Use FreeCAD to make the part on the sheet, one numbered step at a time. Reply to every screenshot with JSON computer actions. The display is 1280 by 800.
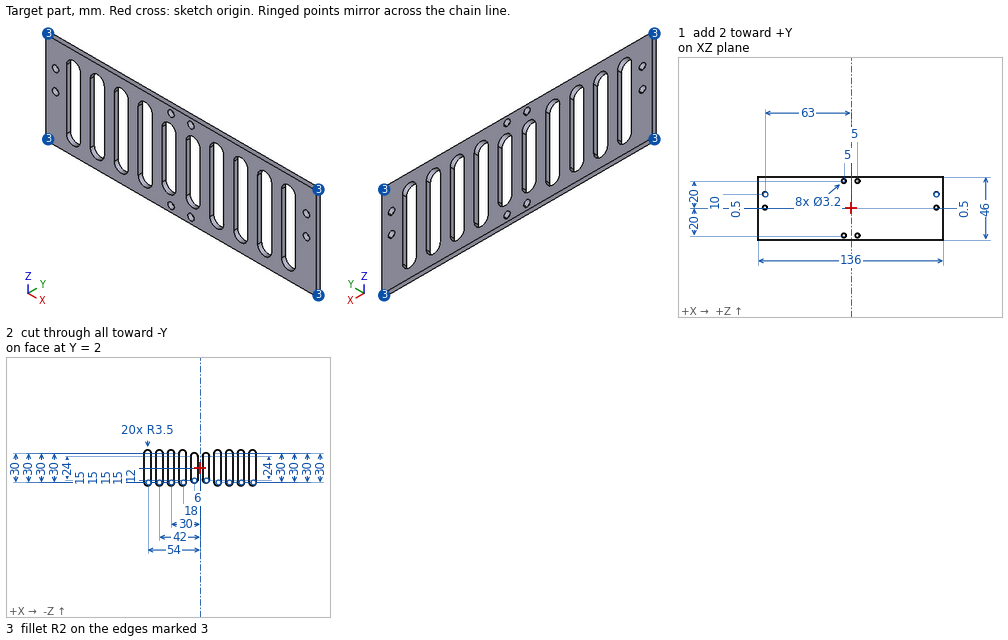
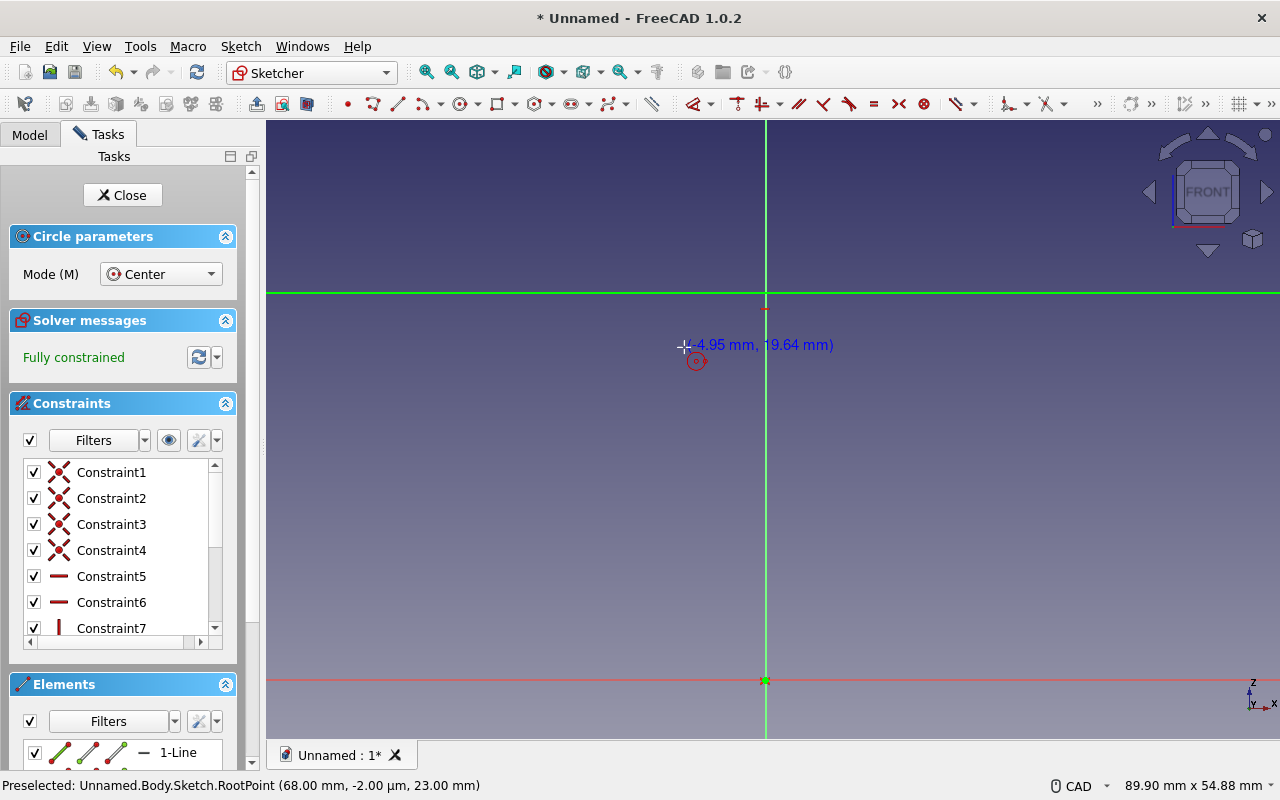
{"action": "scroll", "coordinate": [684, 347], "scroll_direction": "down", "scroll_amount": 7}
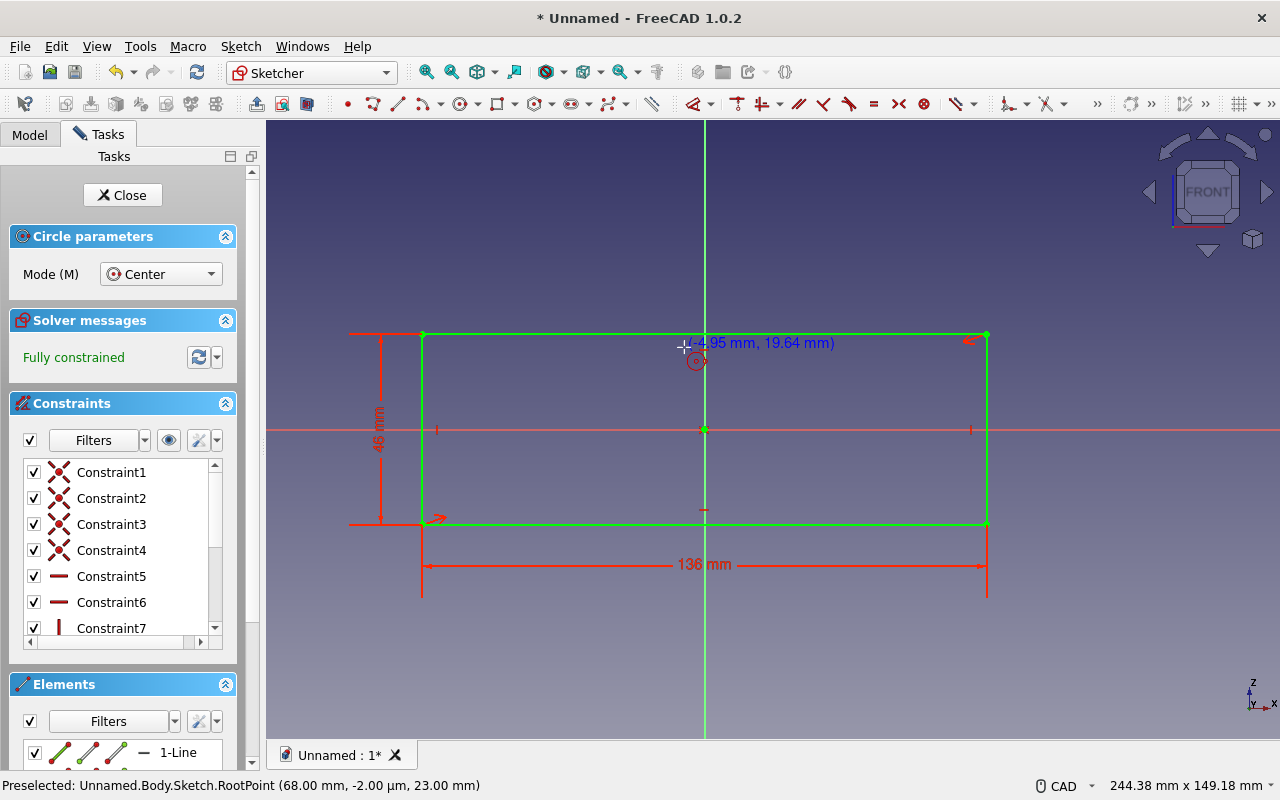
{"action": "scroll", "coordinate": [684, 347], "scroll_direction": "up", "scroll_amount": 2}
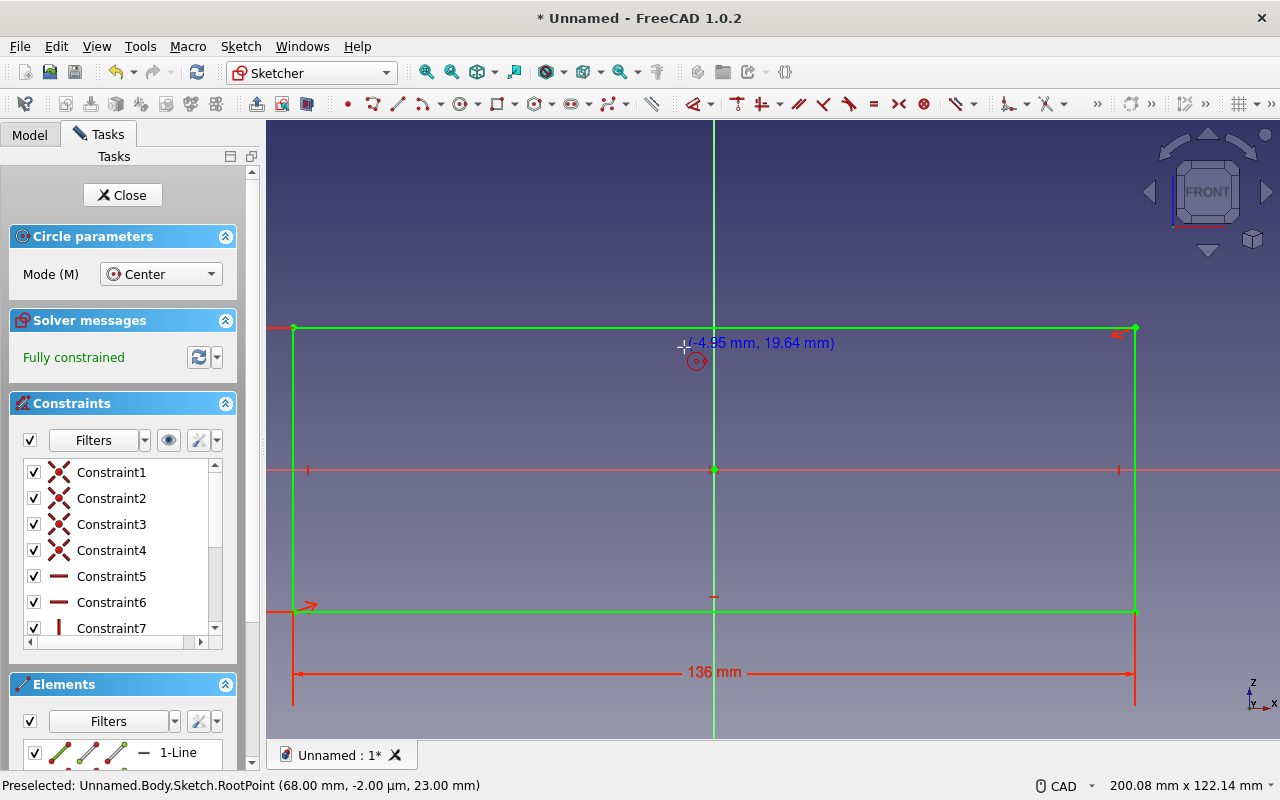
{"action": "left_click", "coordinate": [683, 346]}
{"action": "mouse_move", "coordinate": [690, 353]}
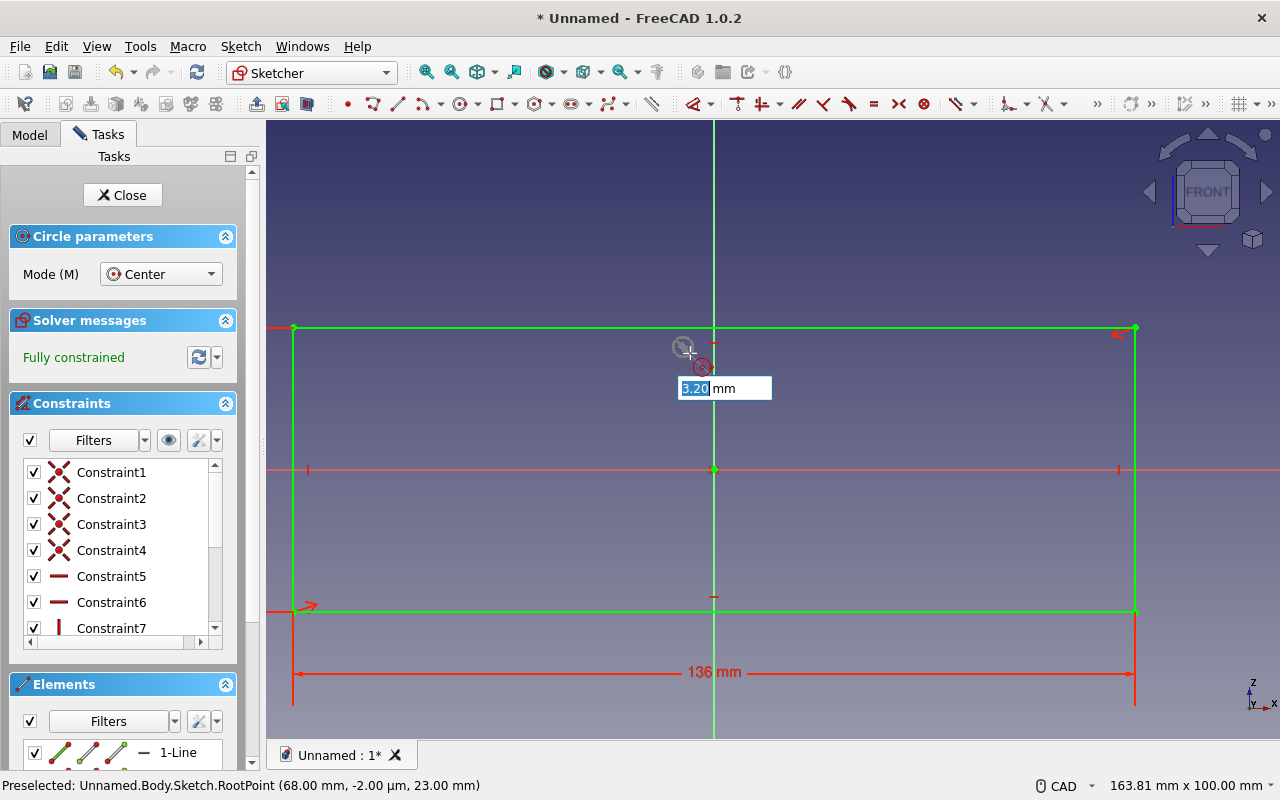
{"action": "type", "text": "3.2"}
{"action": "key", "text": "Return"}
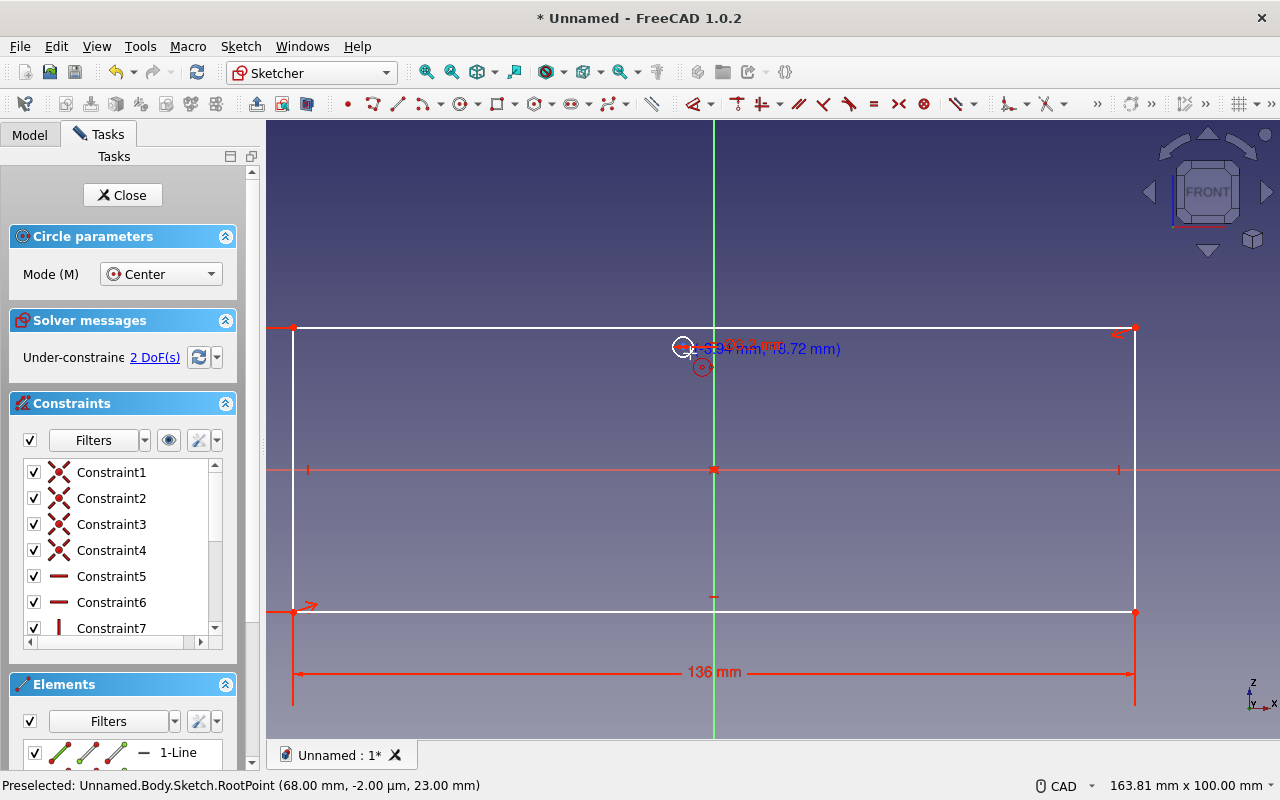
{"action": "scroll", "coordinate": [324, 405], "scroll_direction": "up", "scroll_amount": 5}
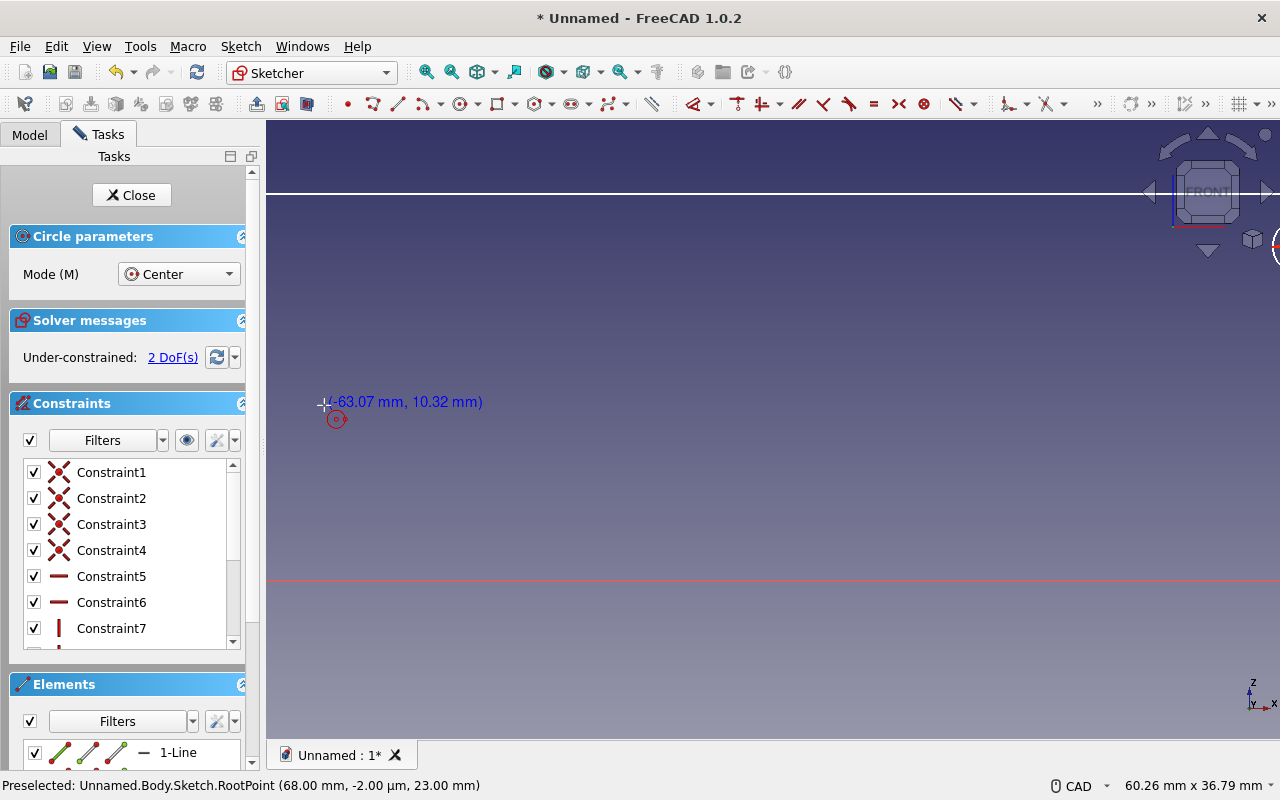
{"action": "scroll", "coordinate": [482, 380], "scroll_direction": "down", "scroll_amount": 7}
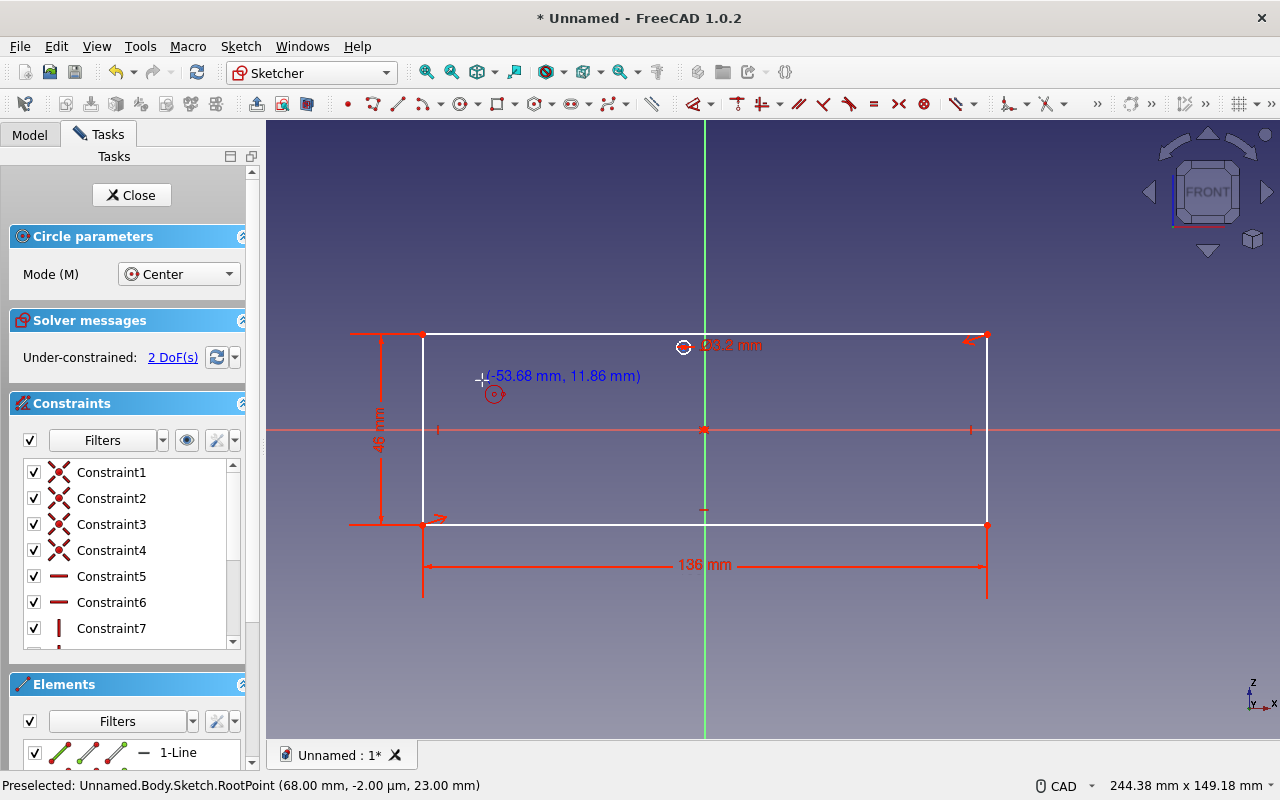
{"action": "left_click", "coordinate": [443, 386]}
{"action": "mouse_move", "coordinate": [448, 382]}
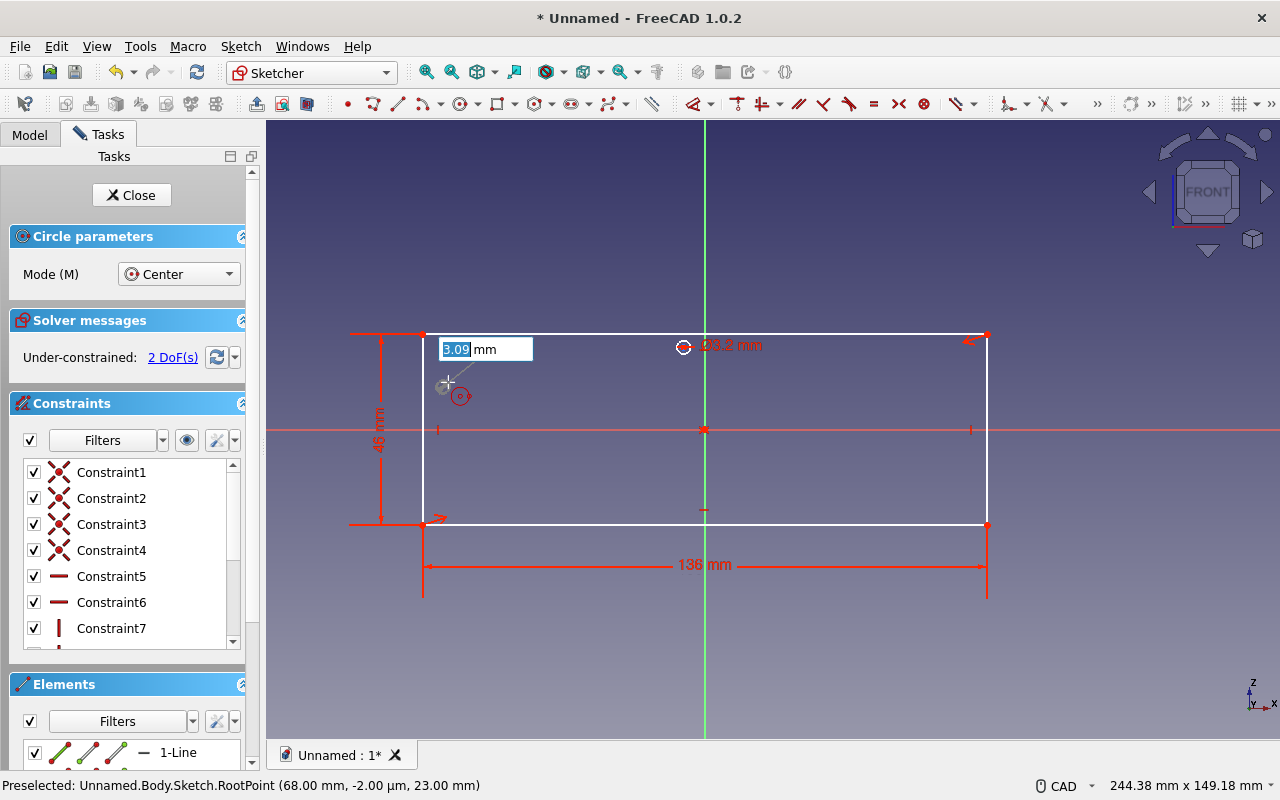
{"action": "type", "text": "3.2"}
{"action": "key", "text": "Return"}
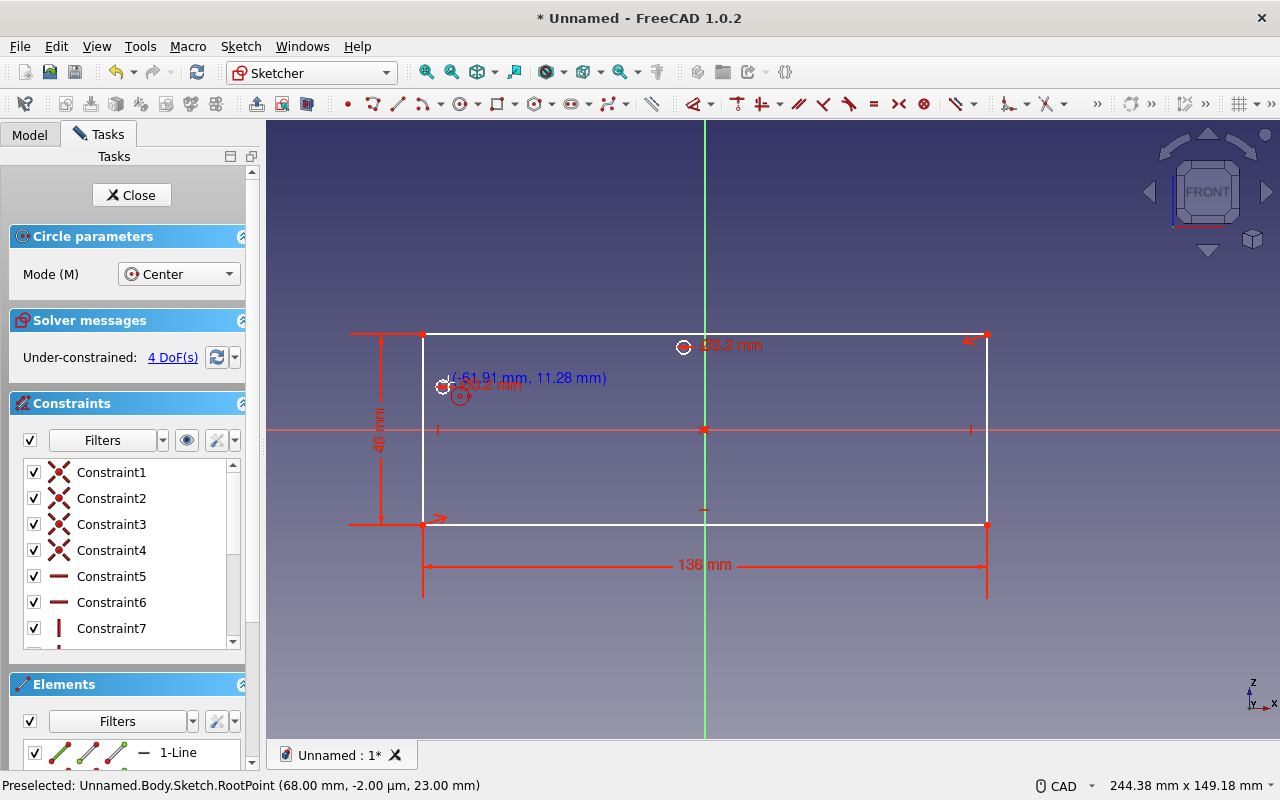
{"action": "scroll", "coordinate": [443, 428], "scroll_direction": "up", "scroll_amount": 11}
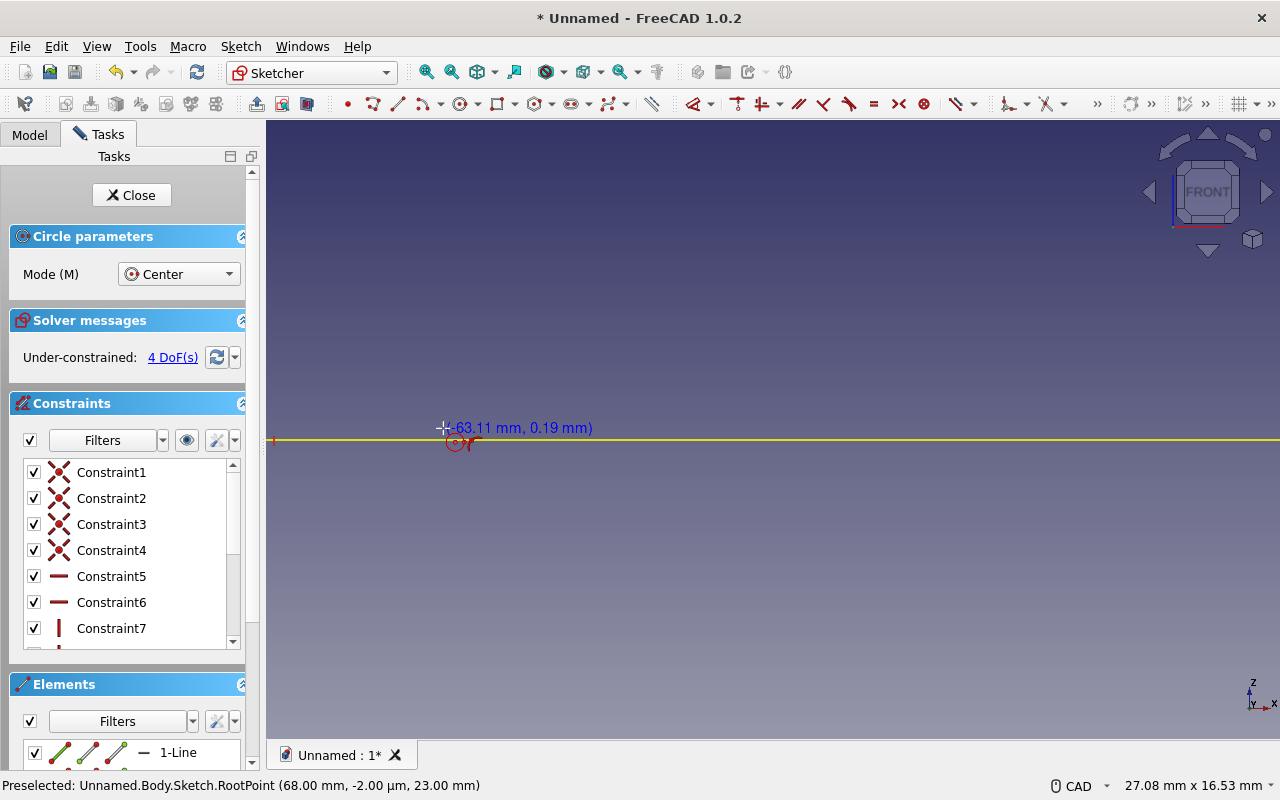
{"action": "left_click", "coordinate": [446, 421]}